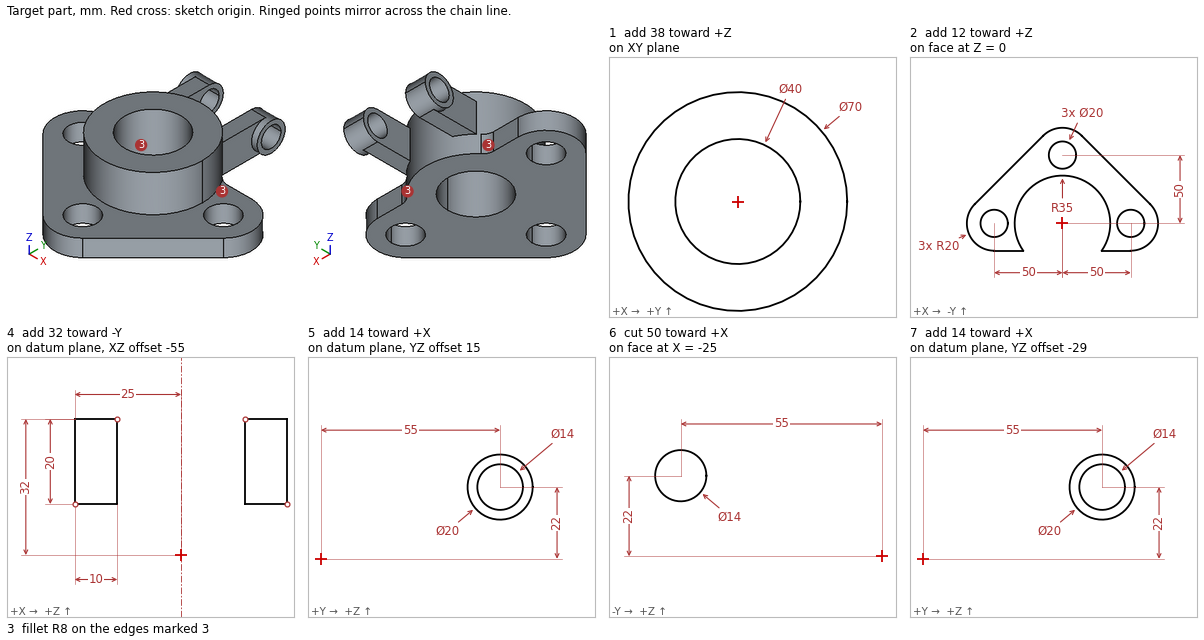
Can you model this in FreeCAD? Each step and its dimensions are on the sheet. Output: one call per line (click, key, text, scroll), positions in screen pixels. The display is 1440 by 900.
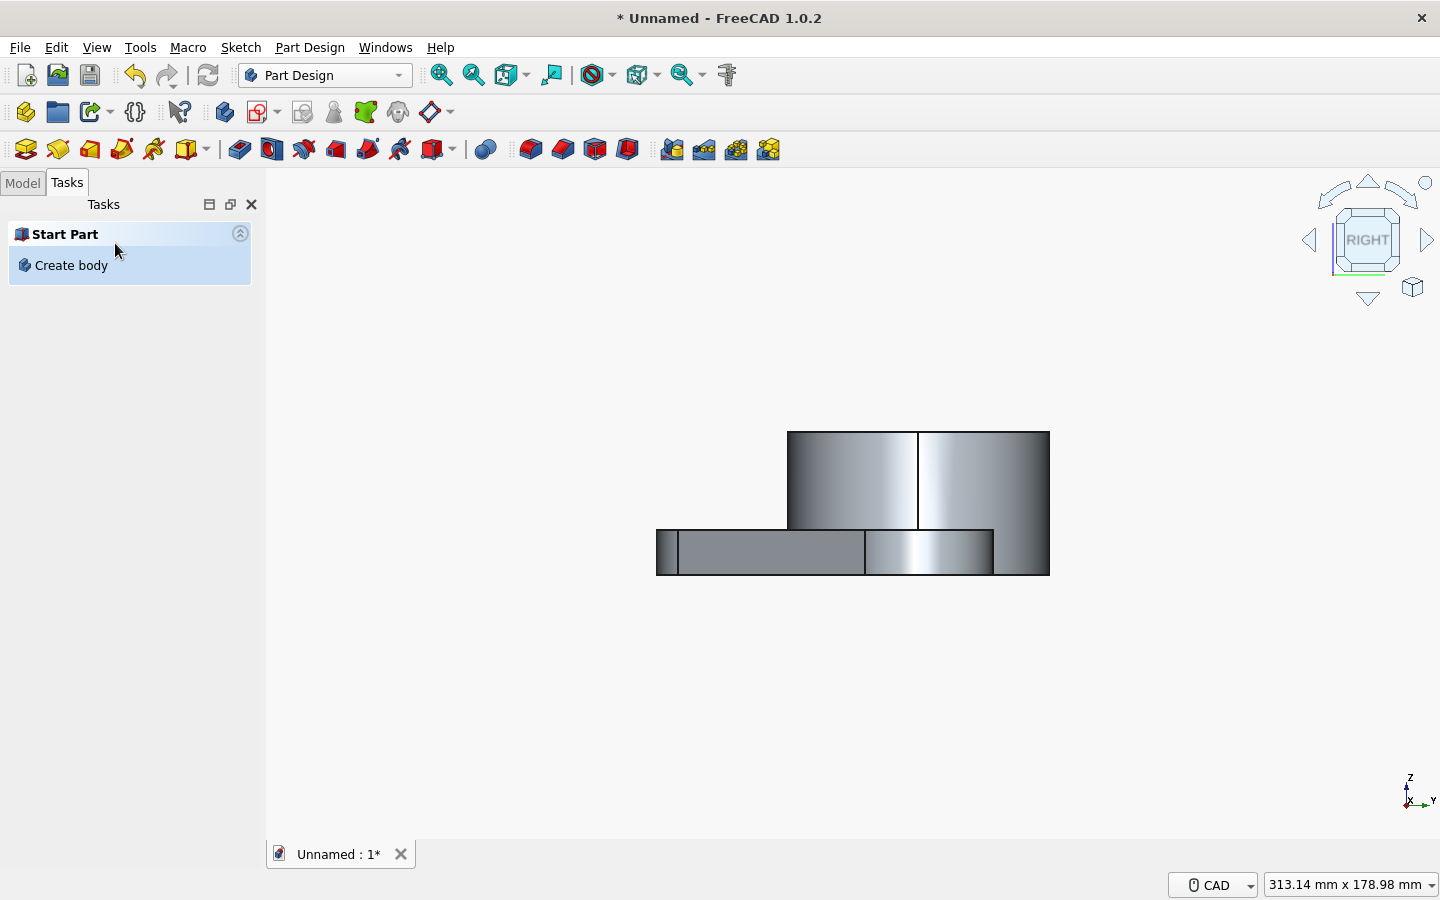
key(v)
key(f)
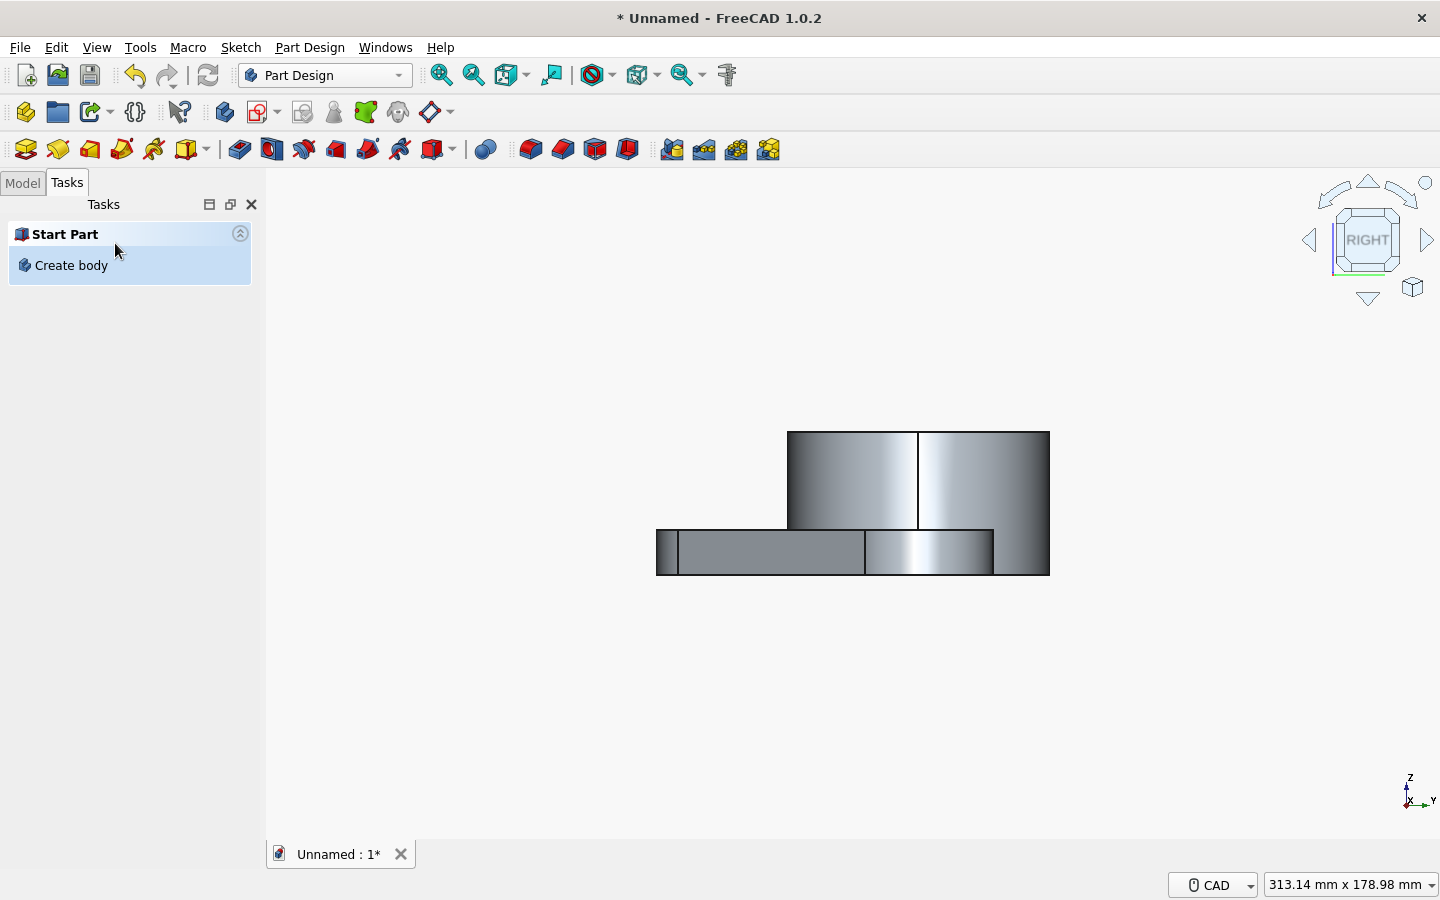
key(5)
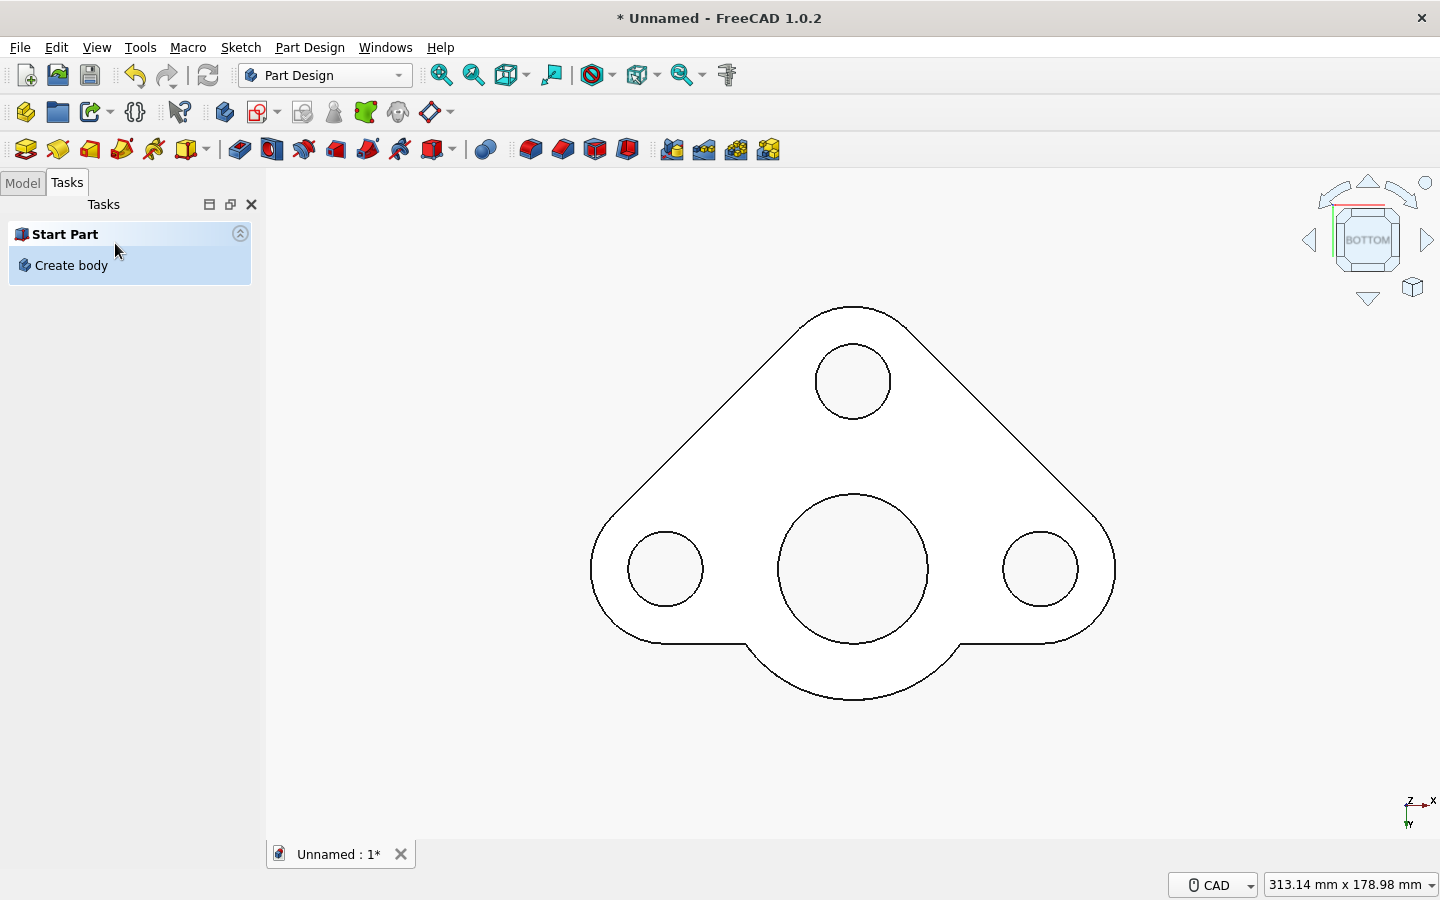
key(4)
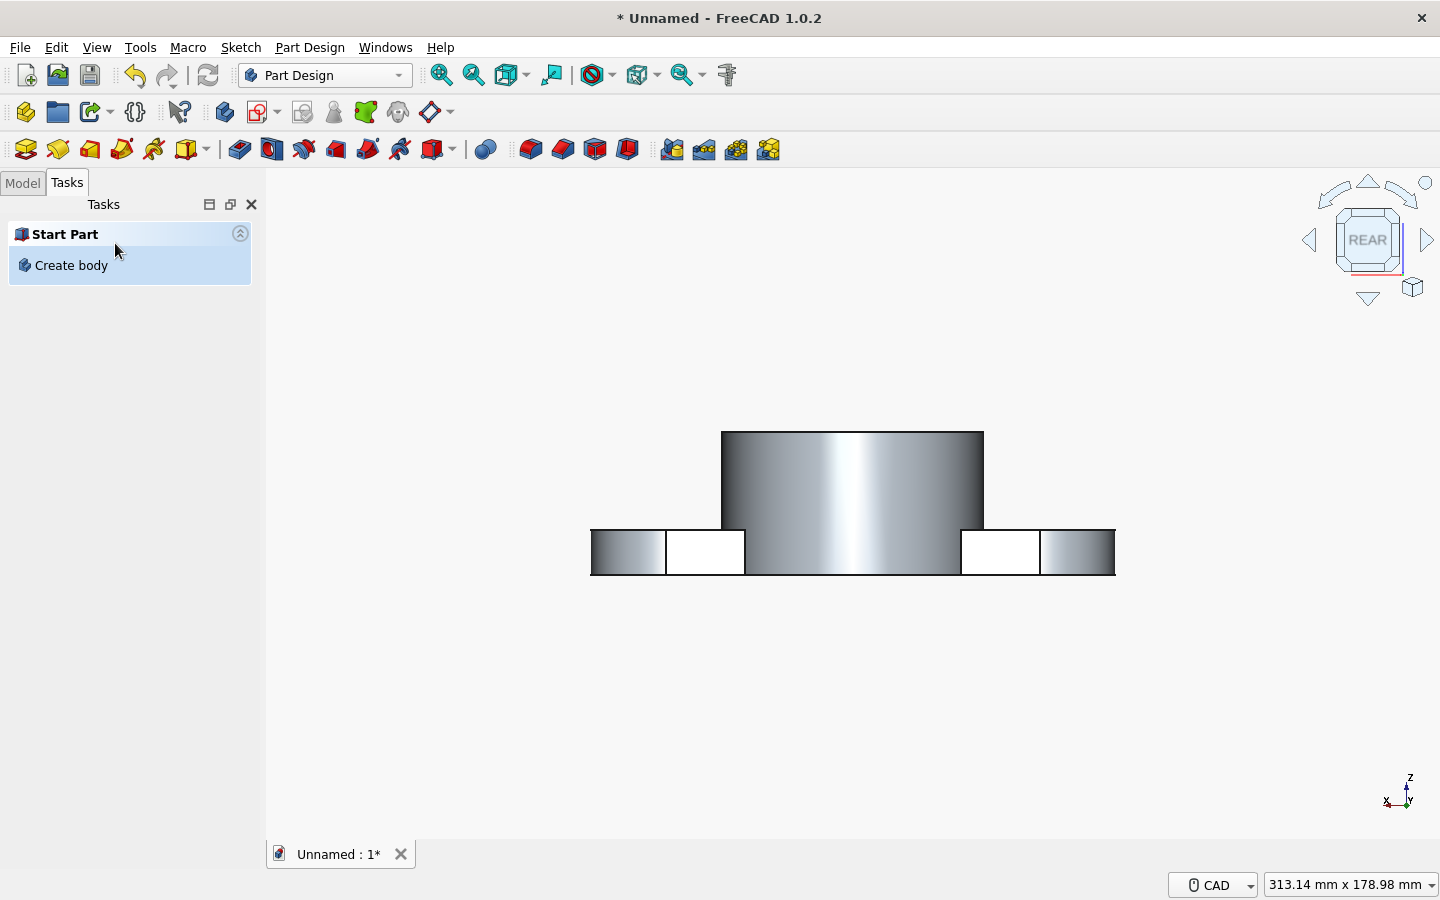
key(v)
key(f)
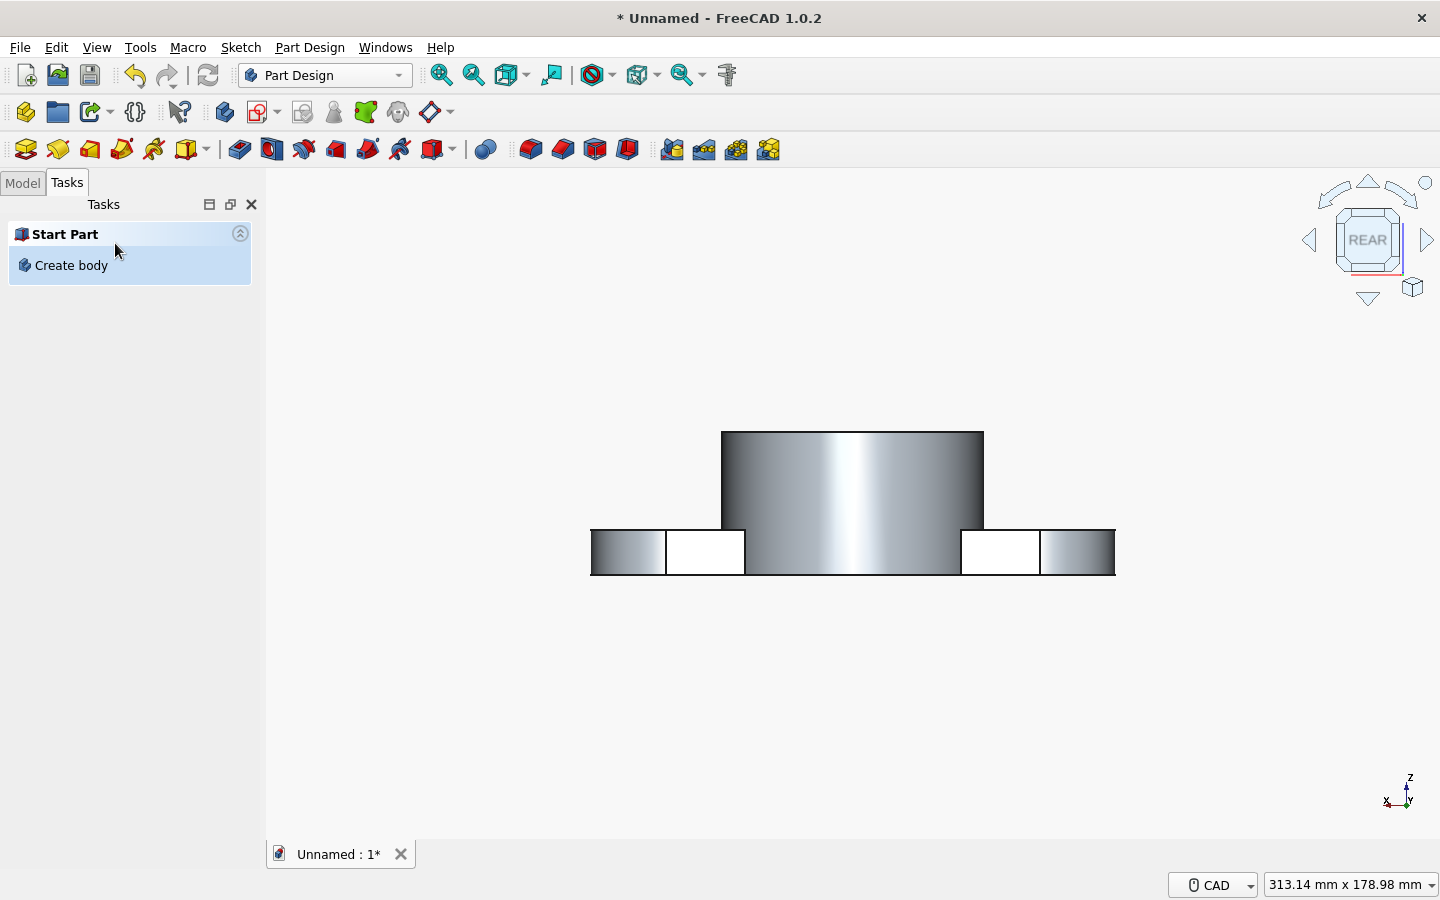
key(6)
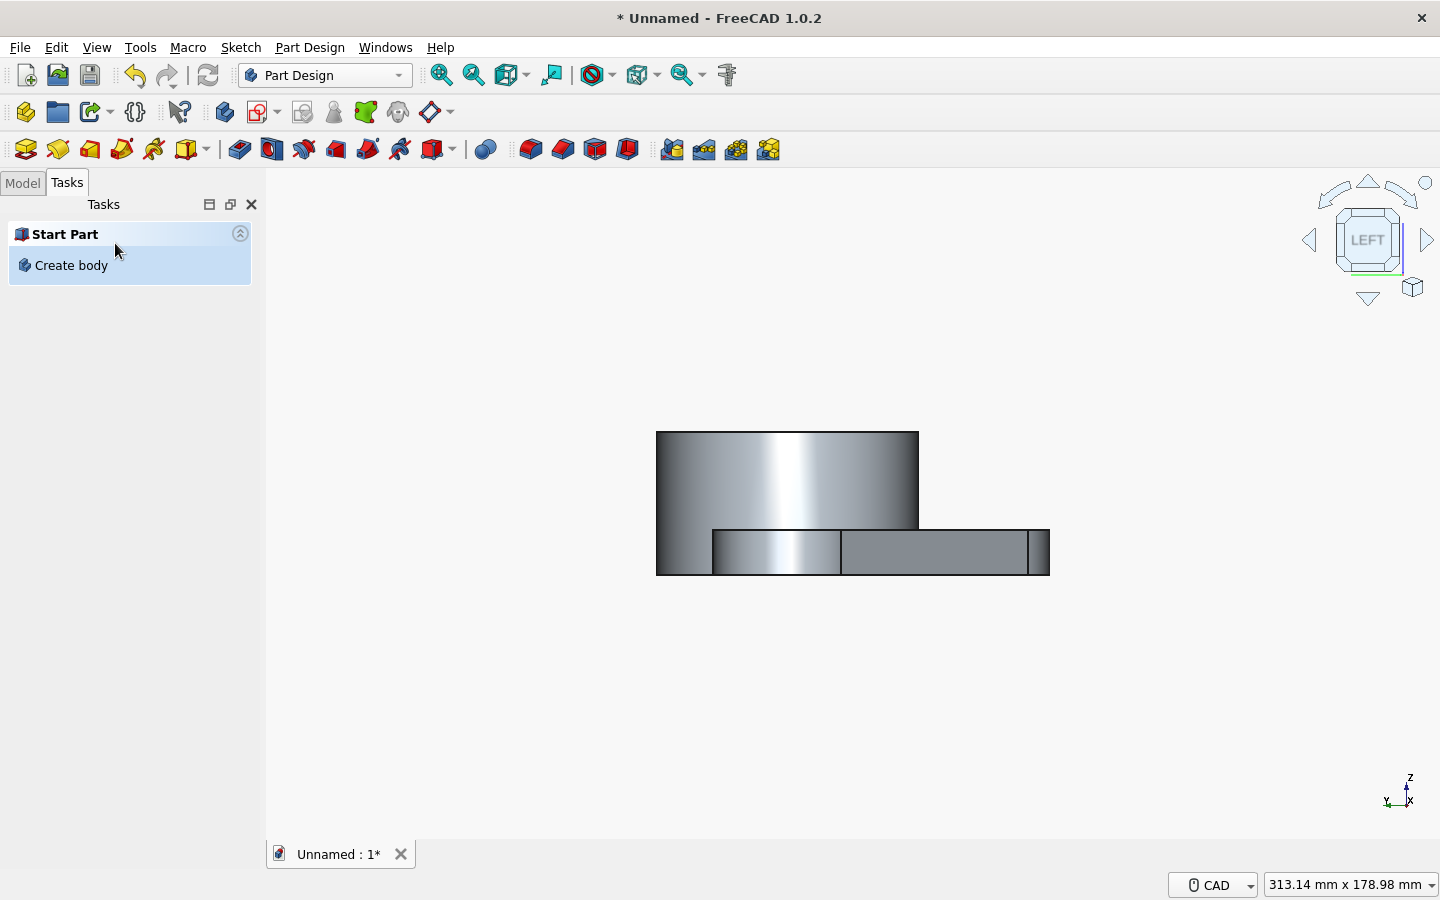
click(442, 76)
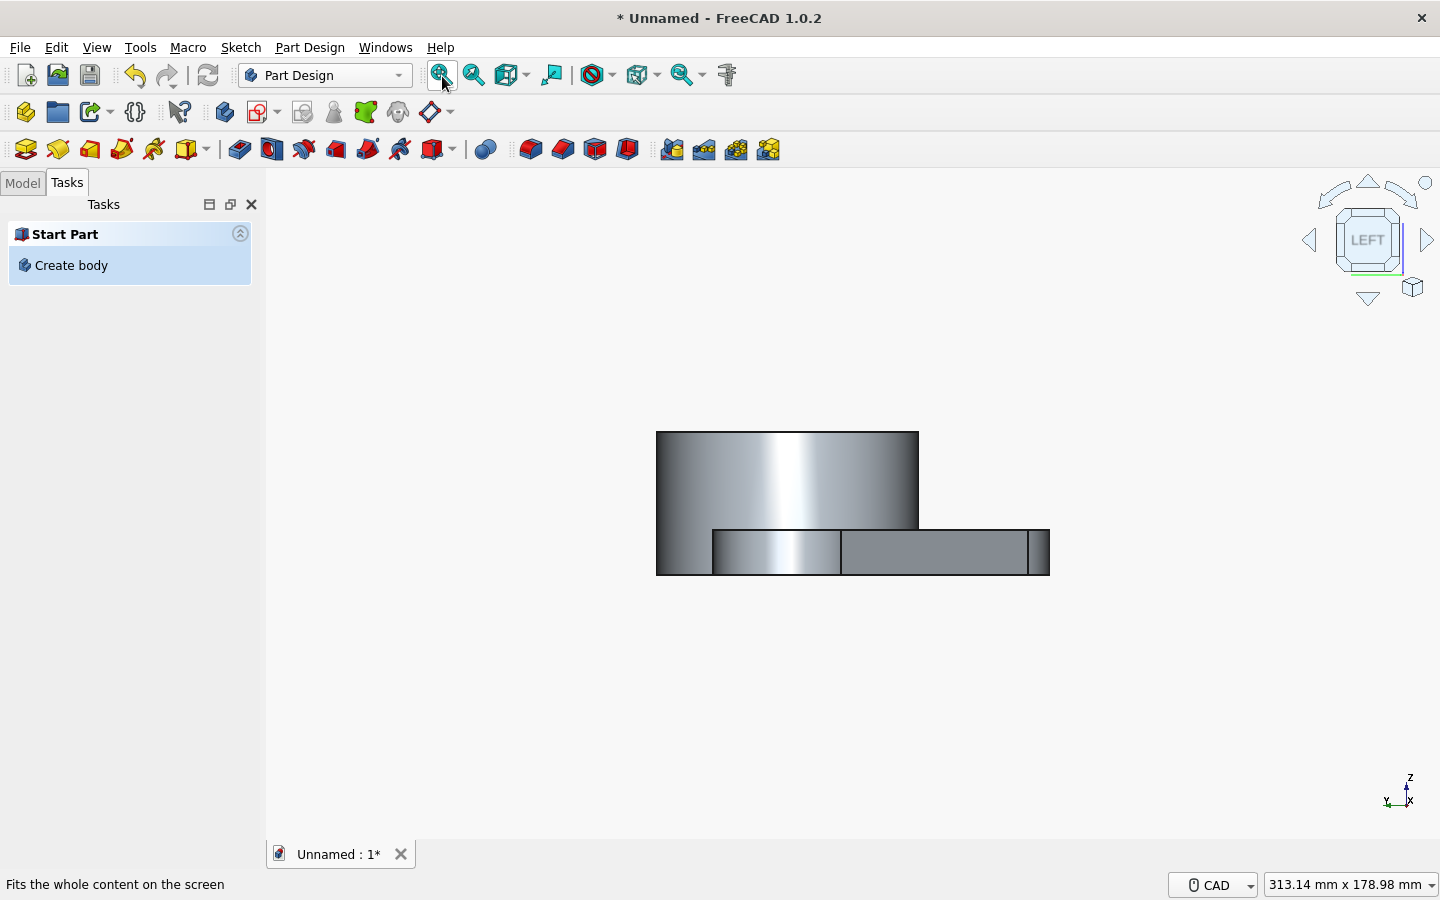
key(v)
key(3)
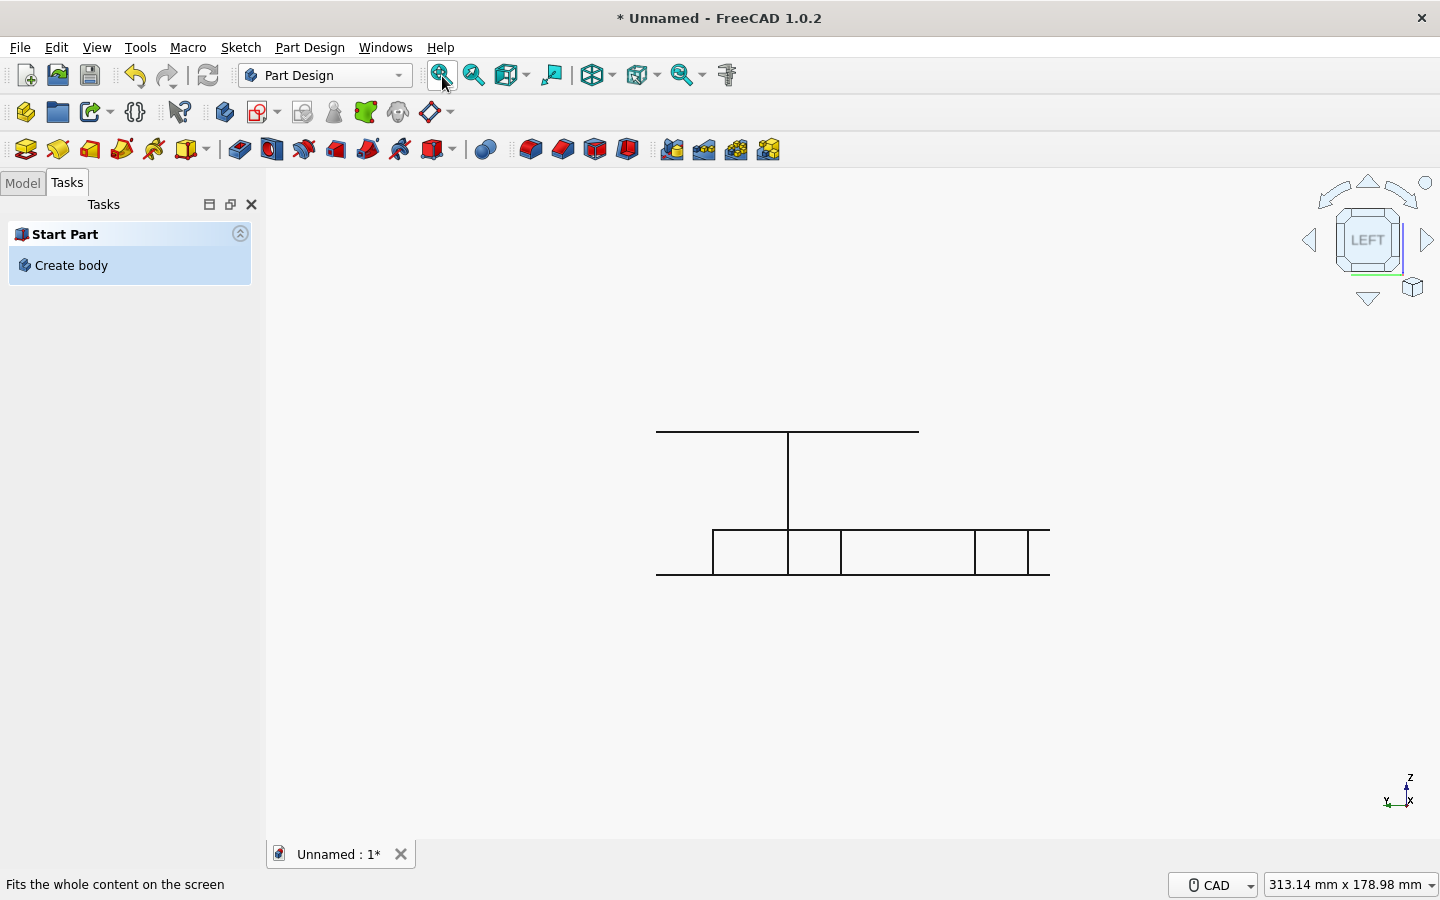
key(0)